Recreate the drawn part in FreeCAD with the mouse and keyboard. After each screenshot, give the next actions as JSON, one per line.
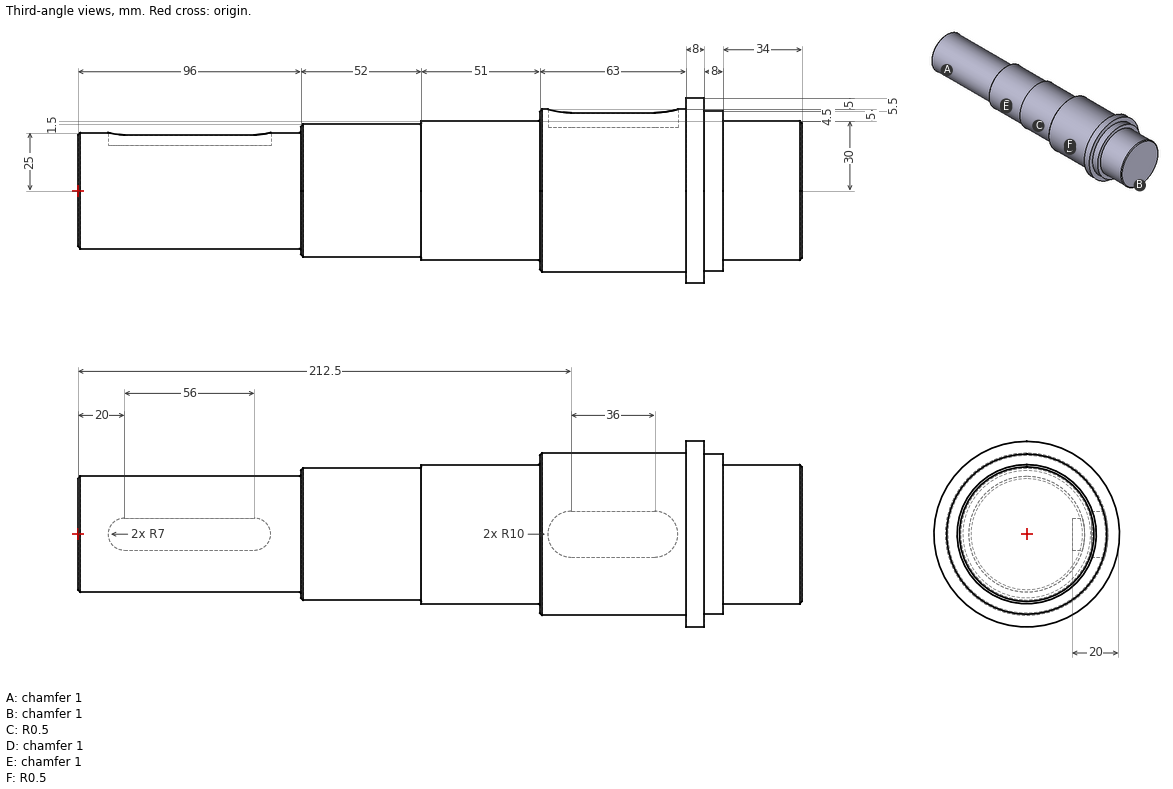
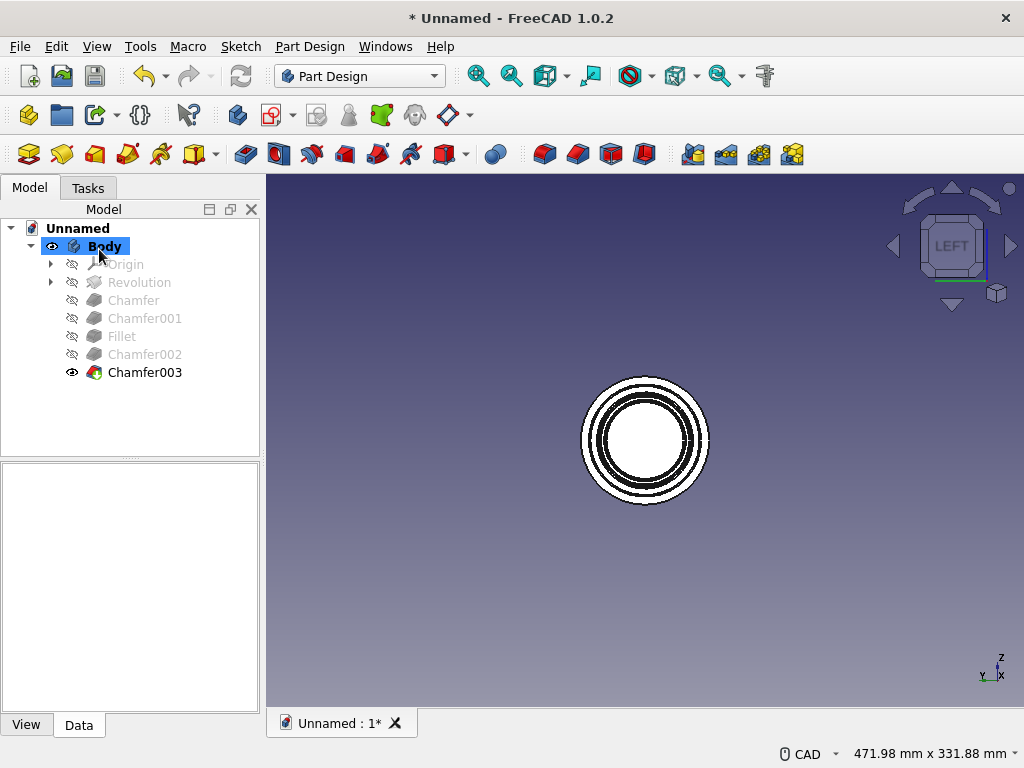
{"action": "key", "text": "v f"}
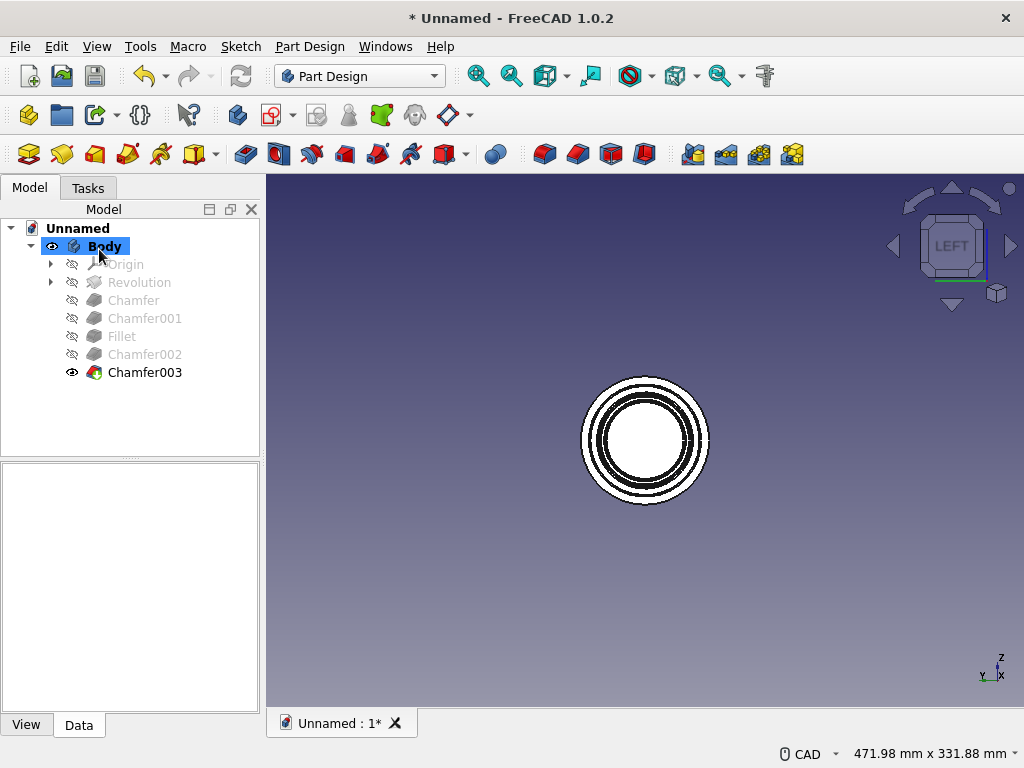
{"action": "key", "text": "v 3"}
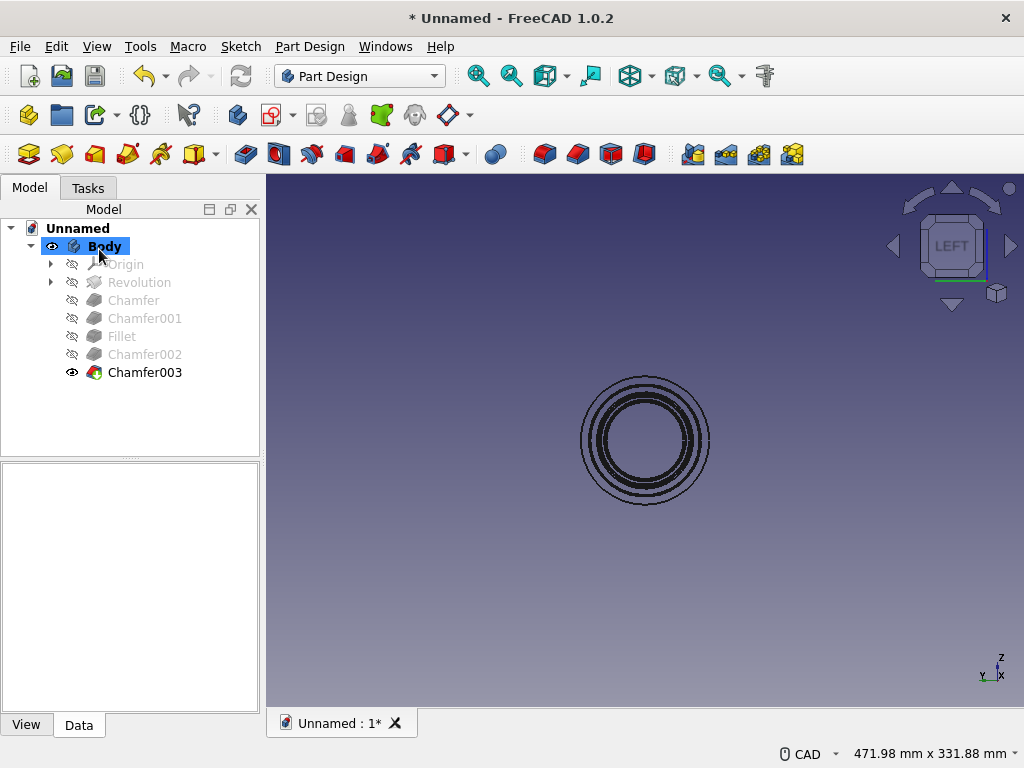
{"action": "key", "text": "0"}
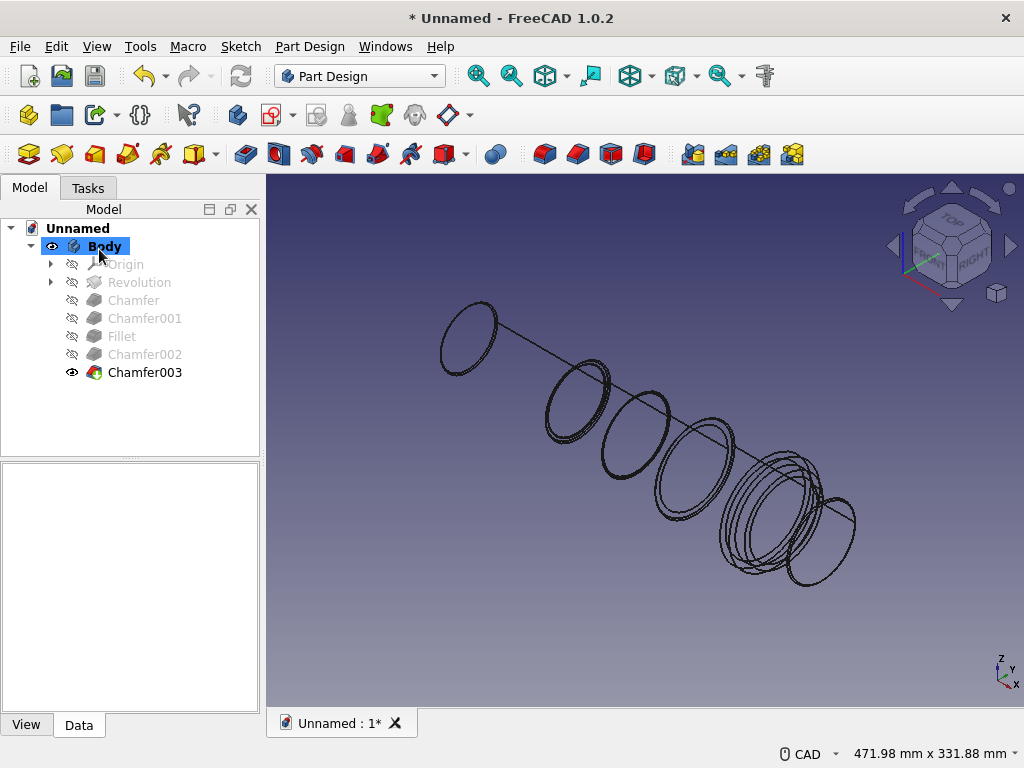
{"action": "left_click", "coordinate": [683, 511]}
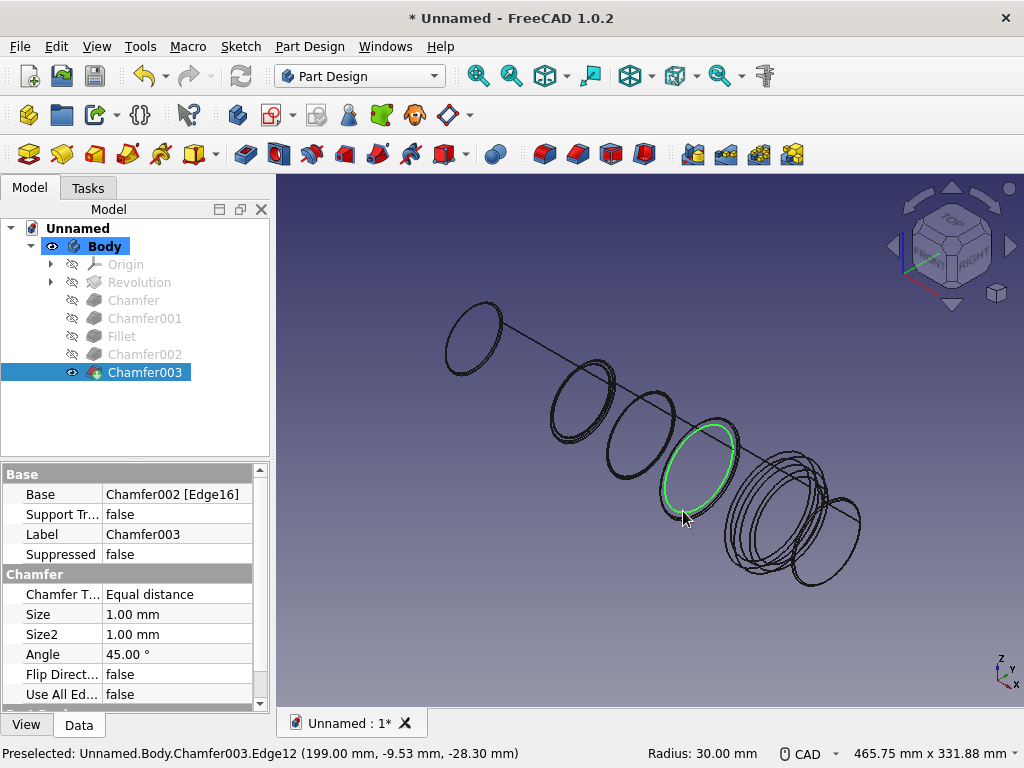
{"action": "key", "text": "v 1"}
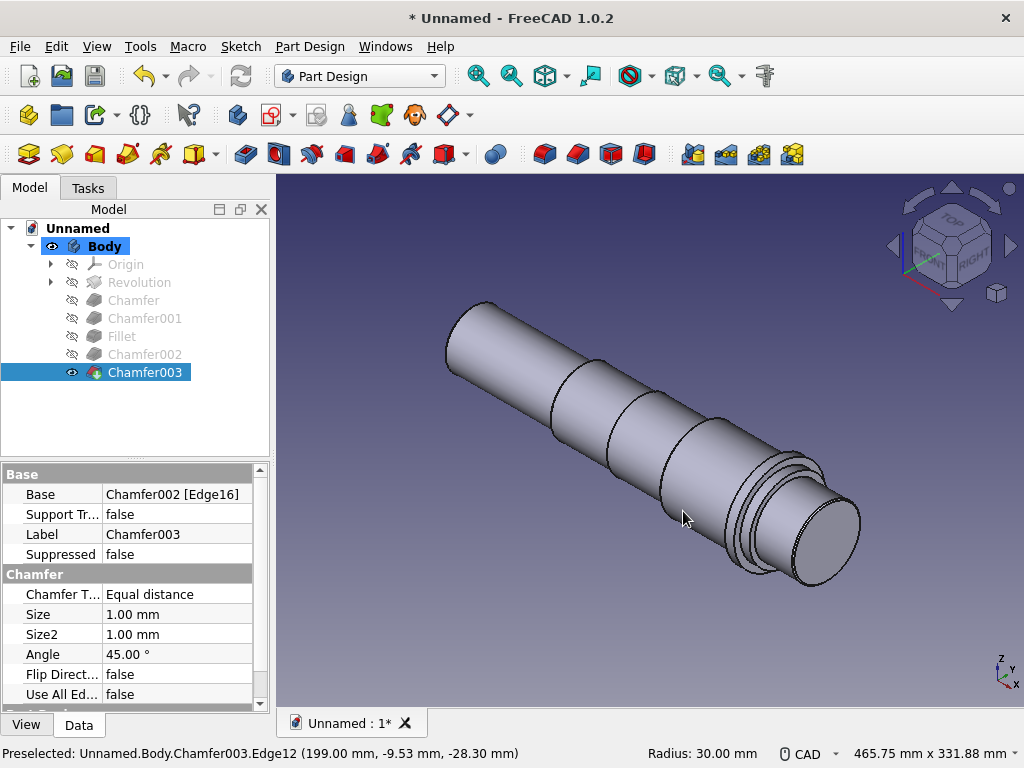
{"action": "left_click", "coordinate": [545, 154]}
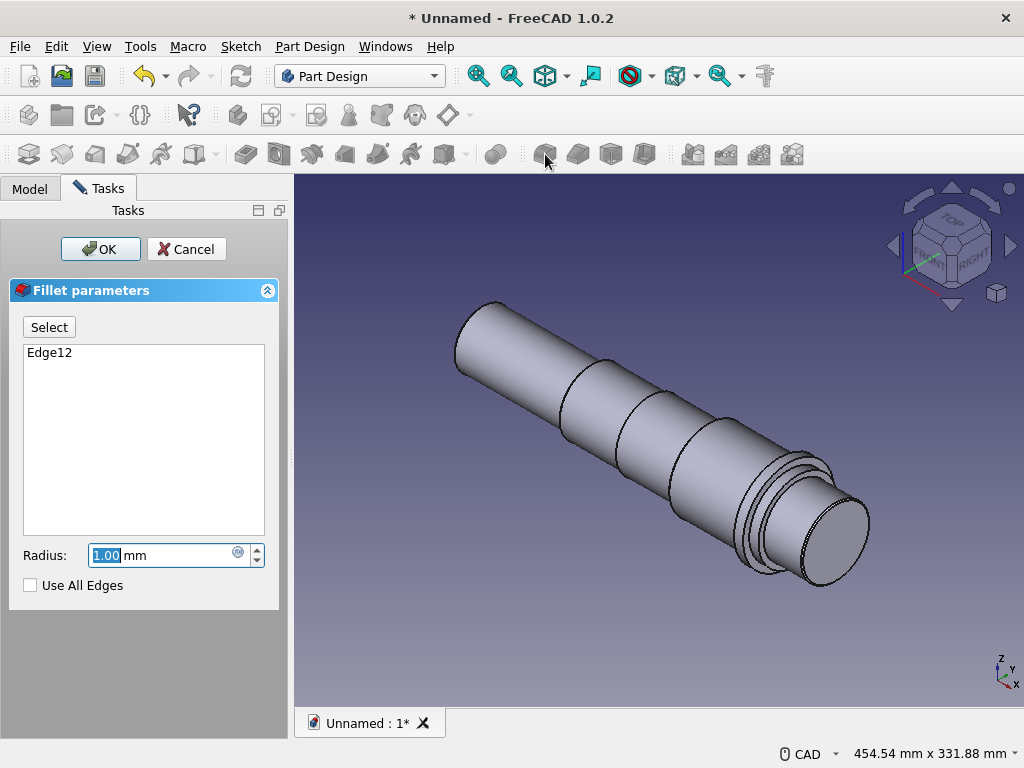
{"action": "type", "text": "0.5"}
{"action": "key", "text": "Tab"}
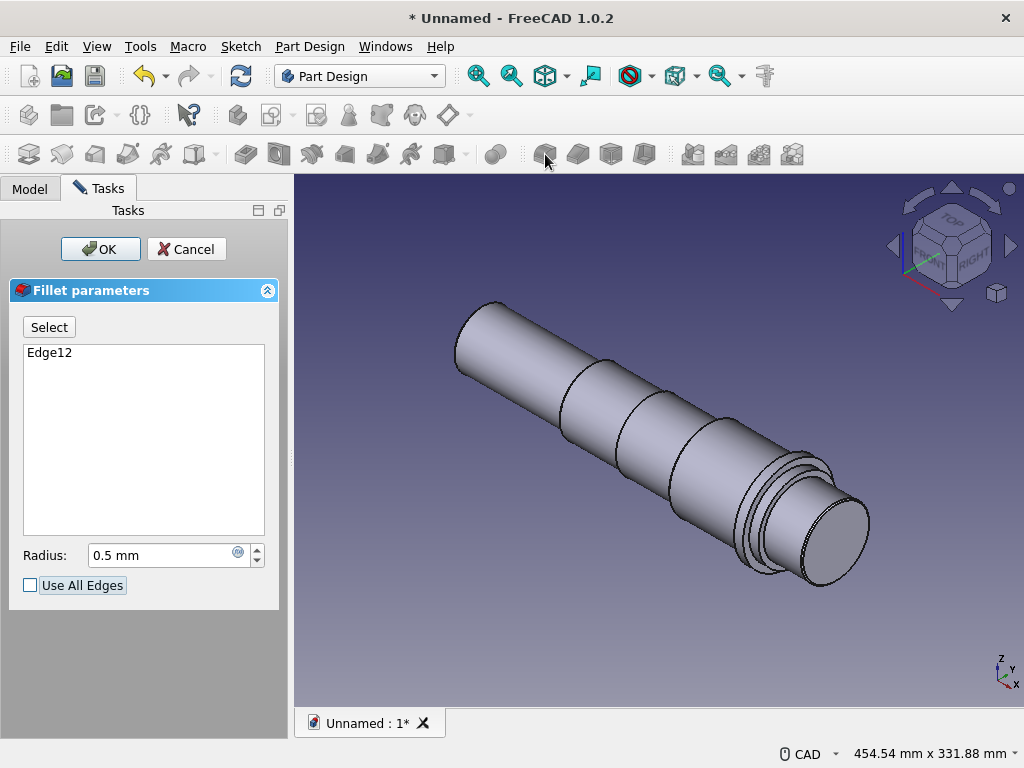
{"action": "left_click", "coordinate": [101, 249]}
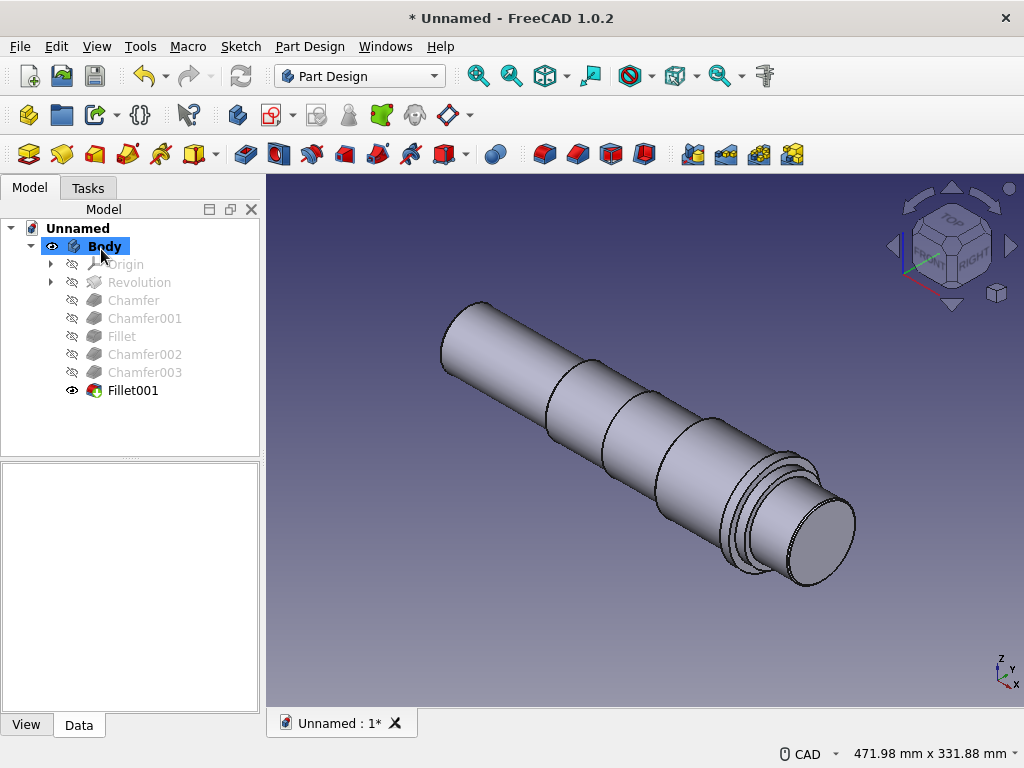
{"action": "left_click", "coordinate": [51, 264]}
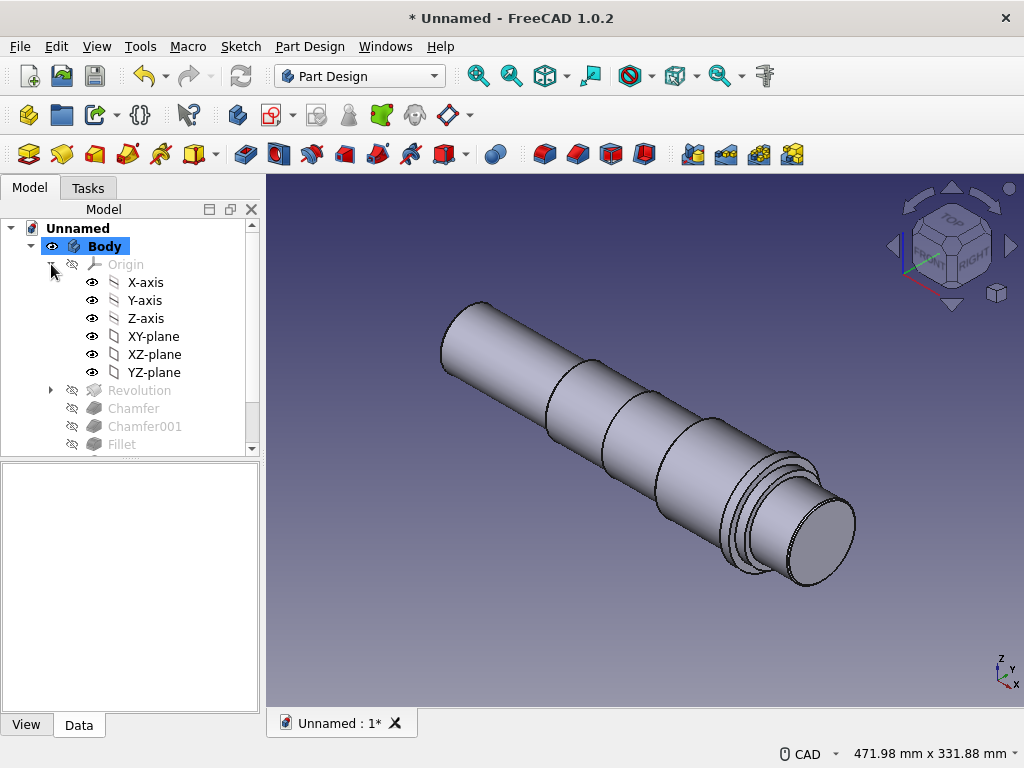
{"action": "left_click", "coordinate": [137, 354]}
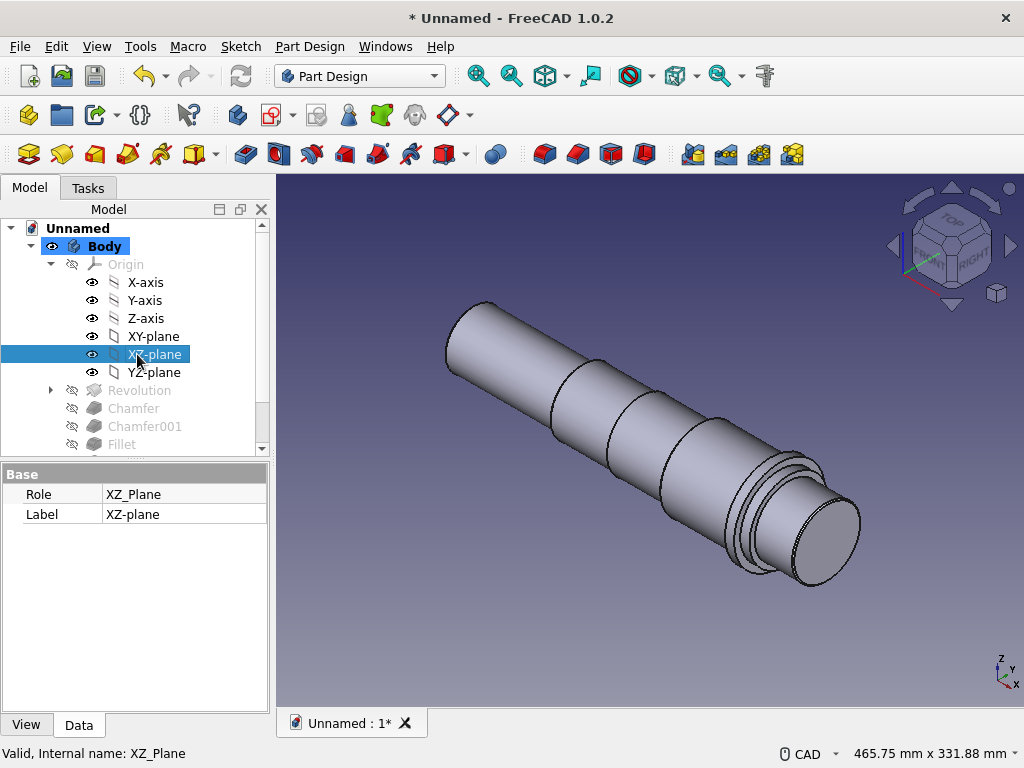
{"action": "left_click", "coordinate": [448, 116]}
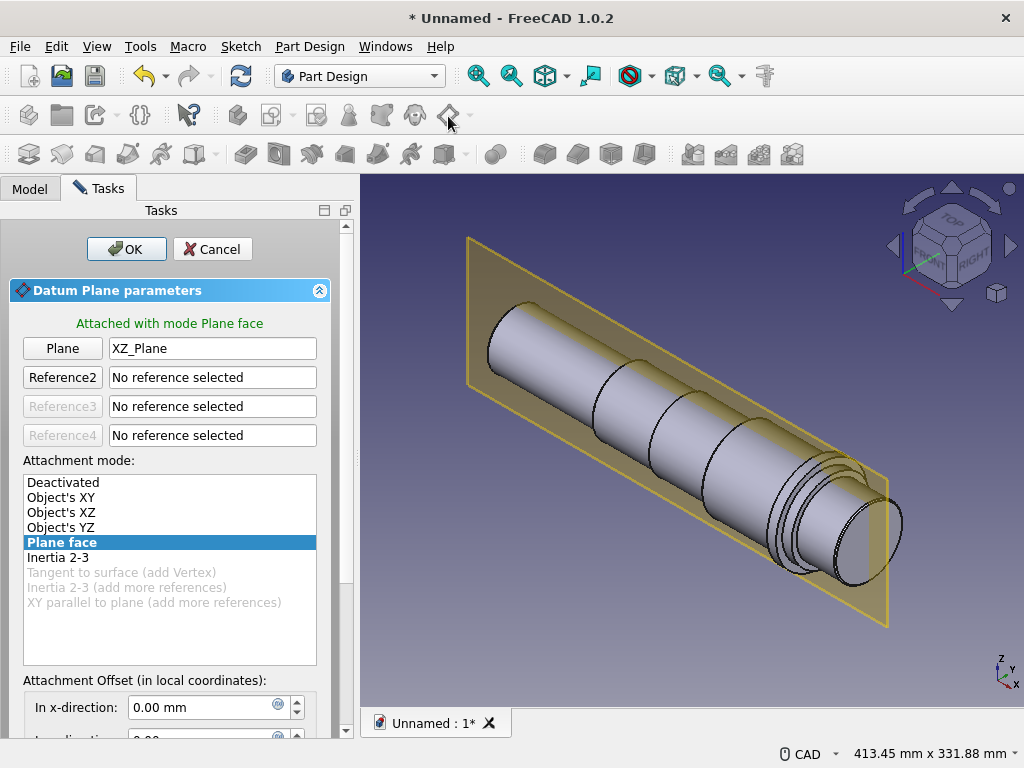
{"action": "scroll", "coordinate": [346, 479], "scroll_direction": "down", "scroll_amount": 2}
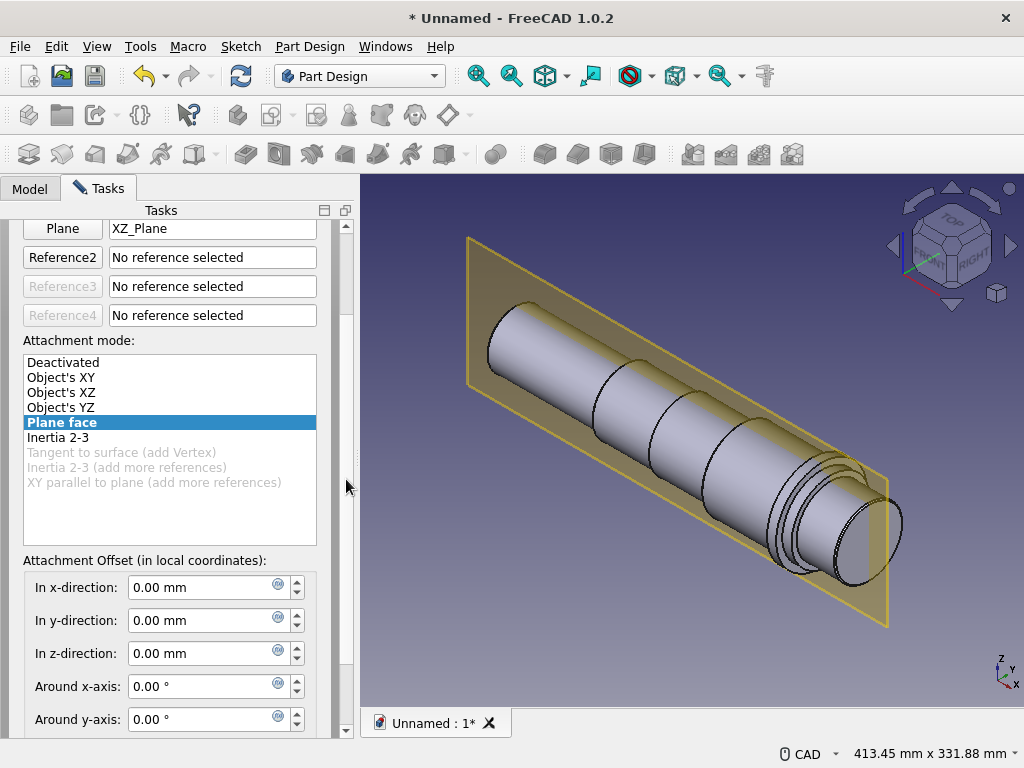
{"action": "triple_click", "coordinate": [210, 654]}